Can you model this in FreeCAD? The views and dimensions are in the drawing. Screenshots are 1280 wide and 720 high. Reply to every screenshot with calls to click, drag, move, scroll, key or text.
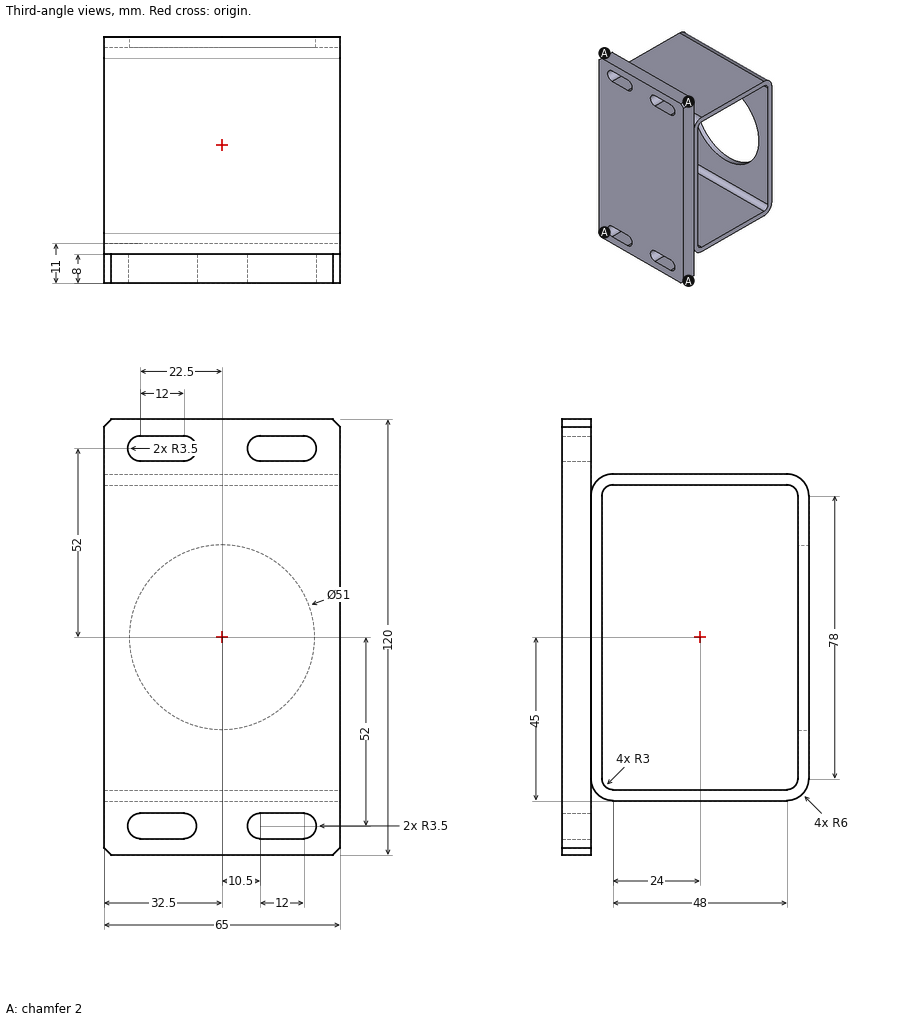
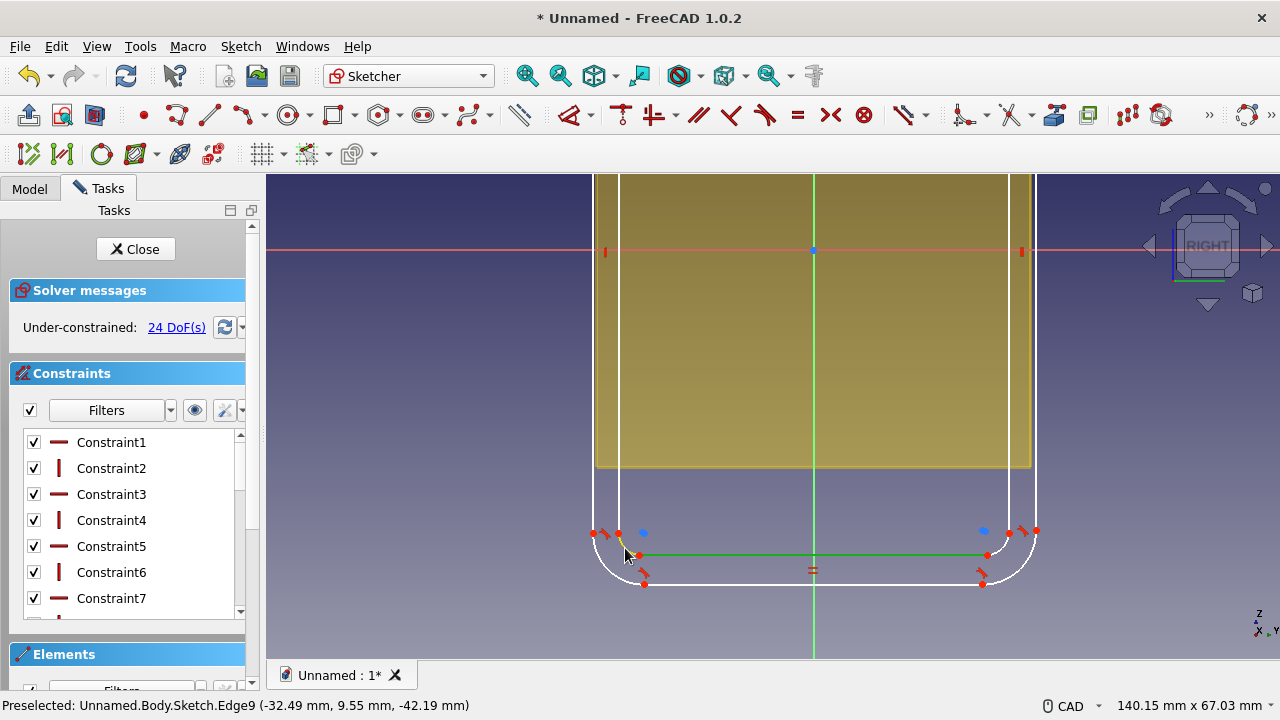
click(625, 548)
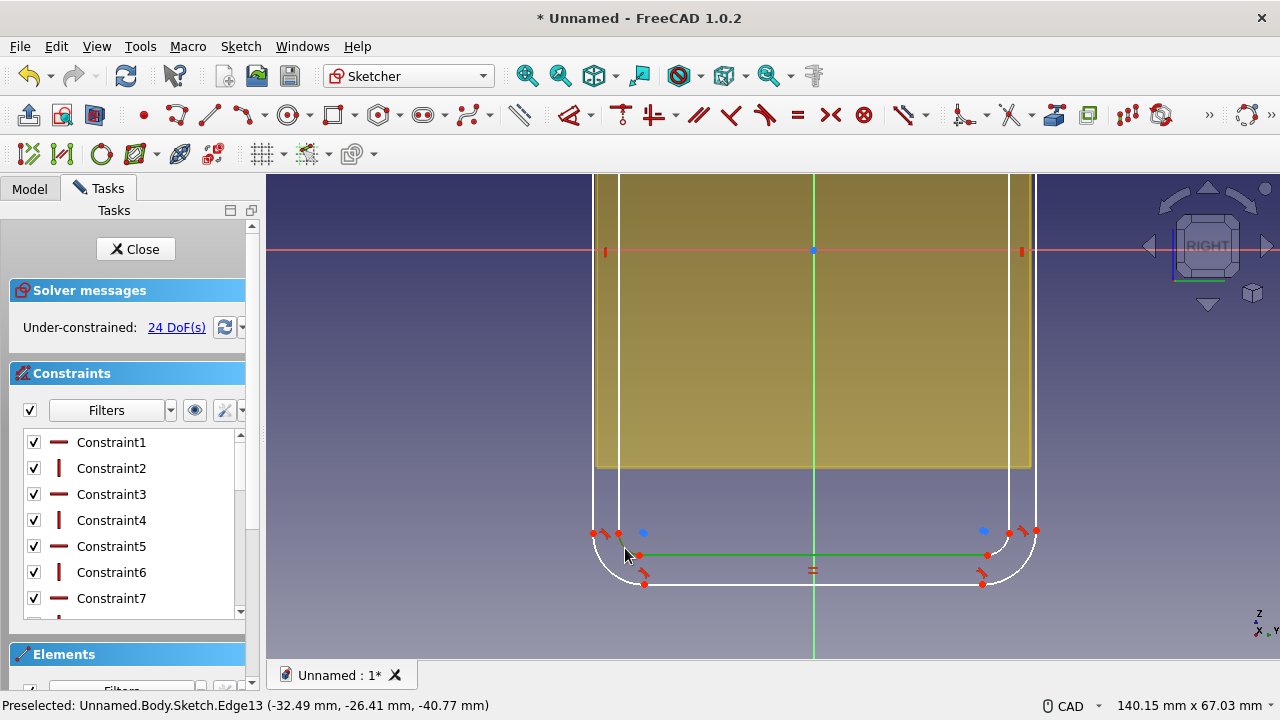
click(765, 116)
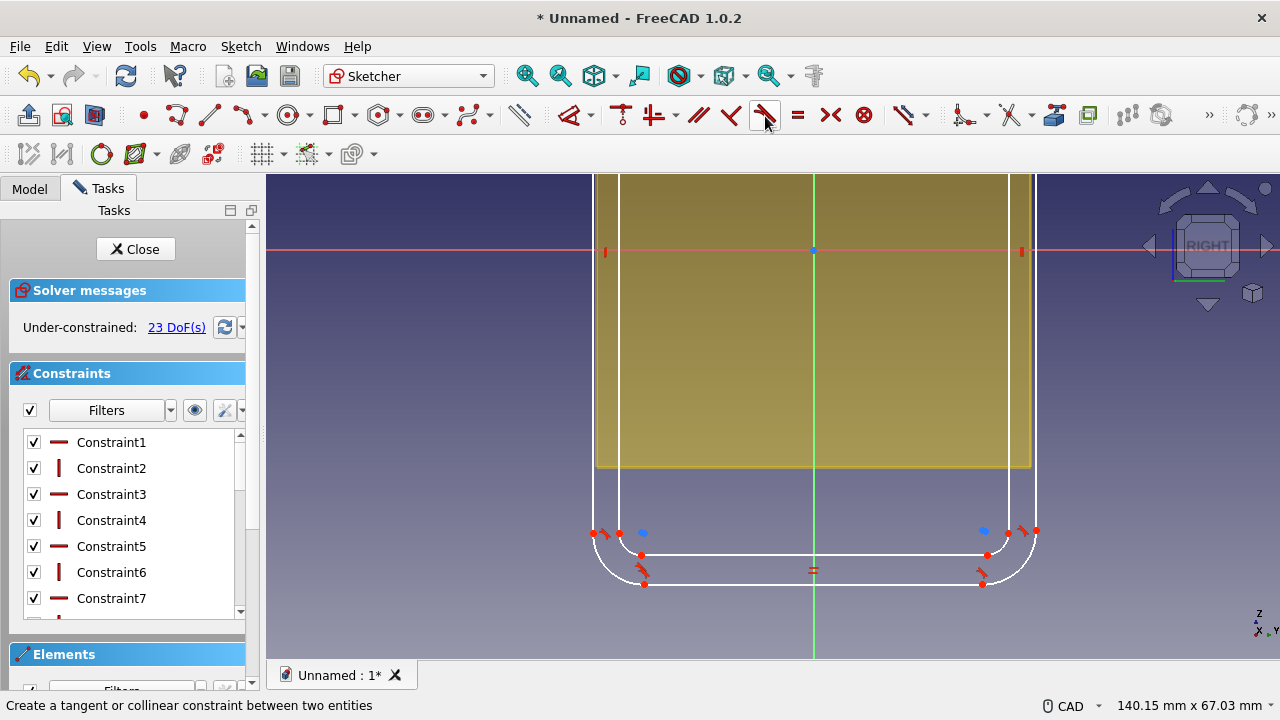
click(884, 555)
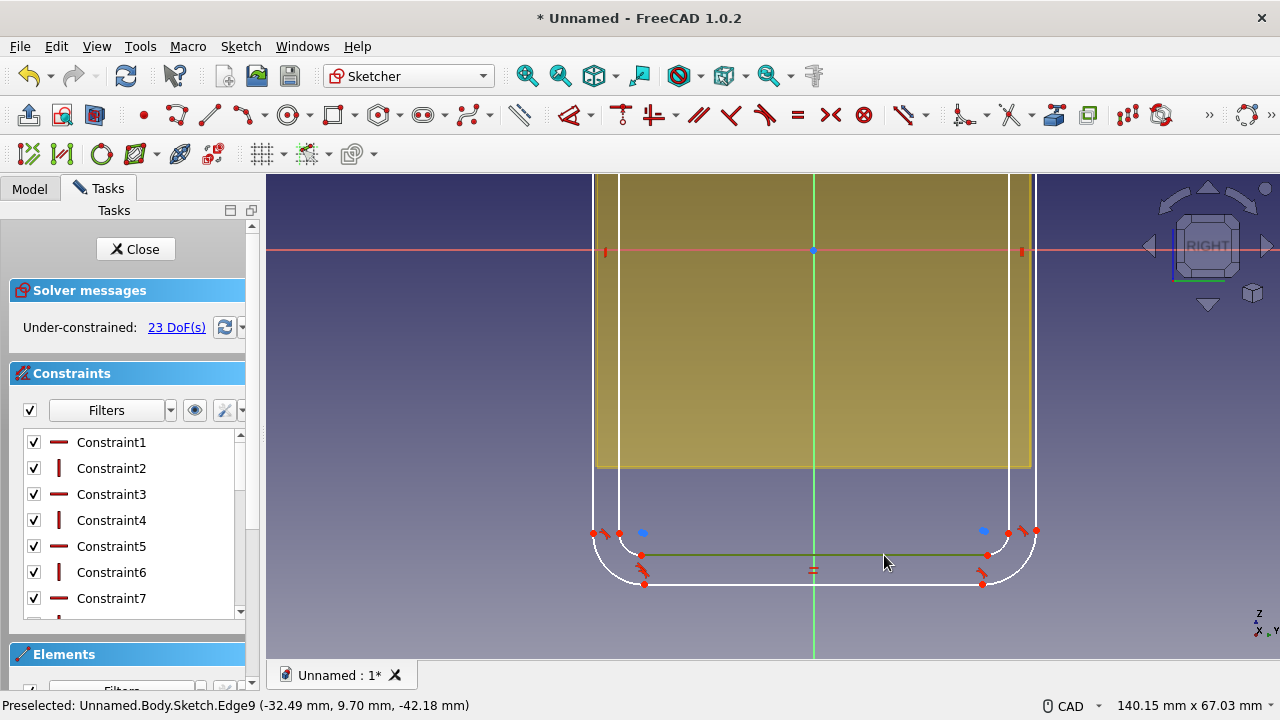
scroll(997, 552, up, 2)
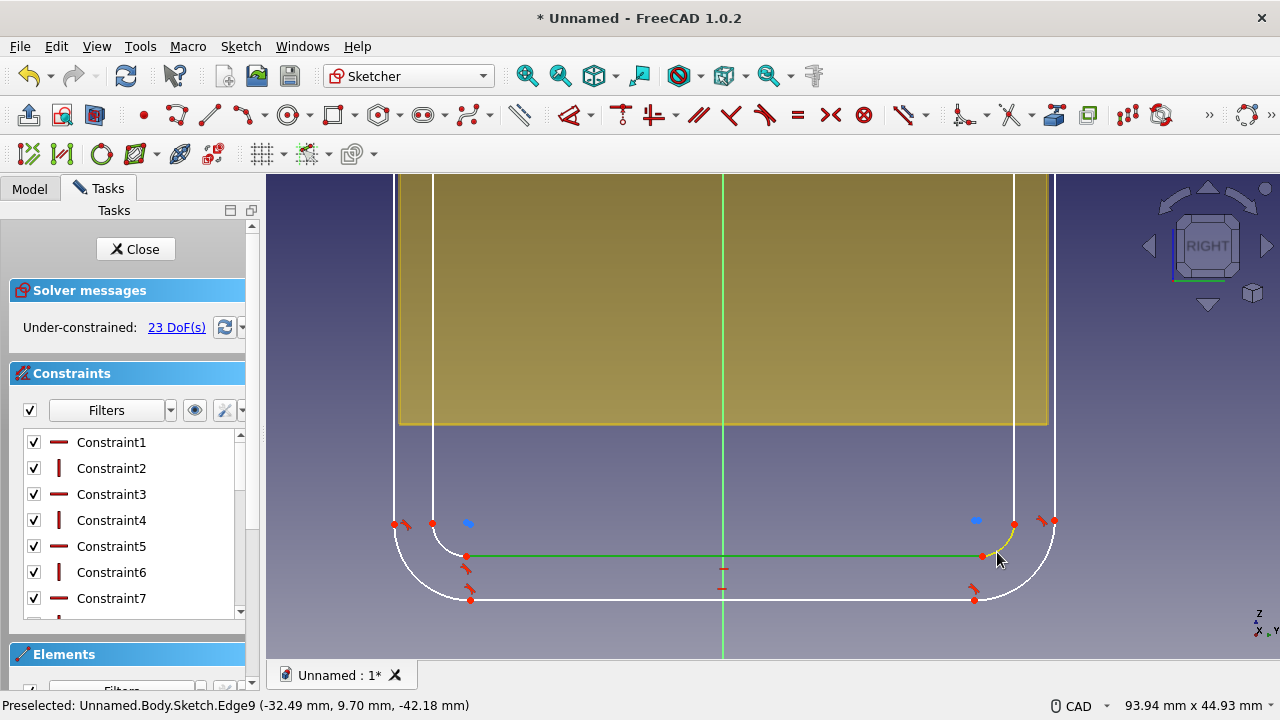
click(997, 552)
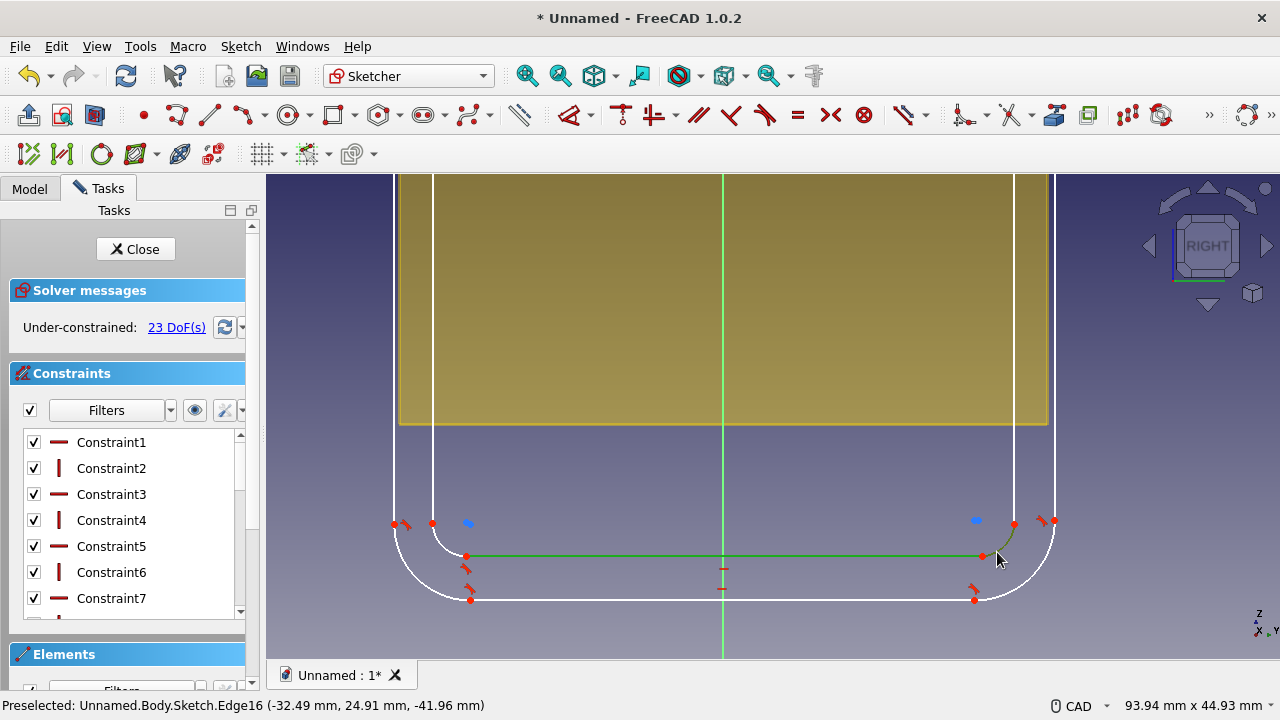
click(765, 116)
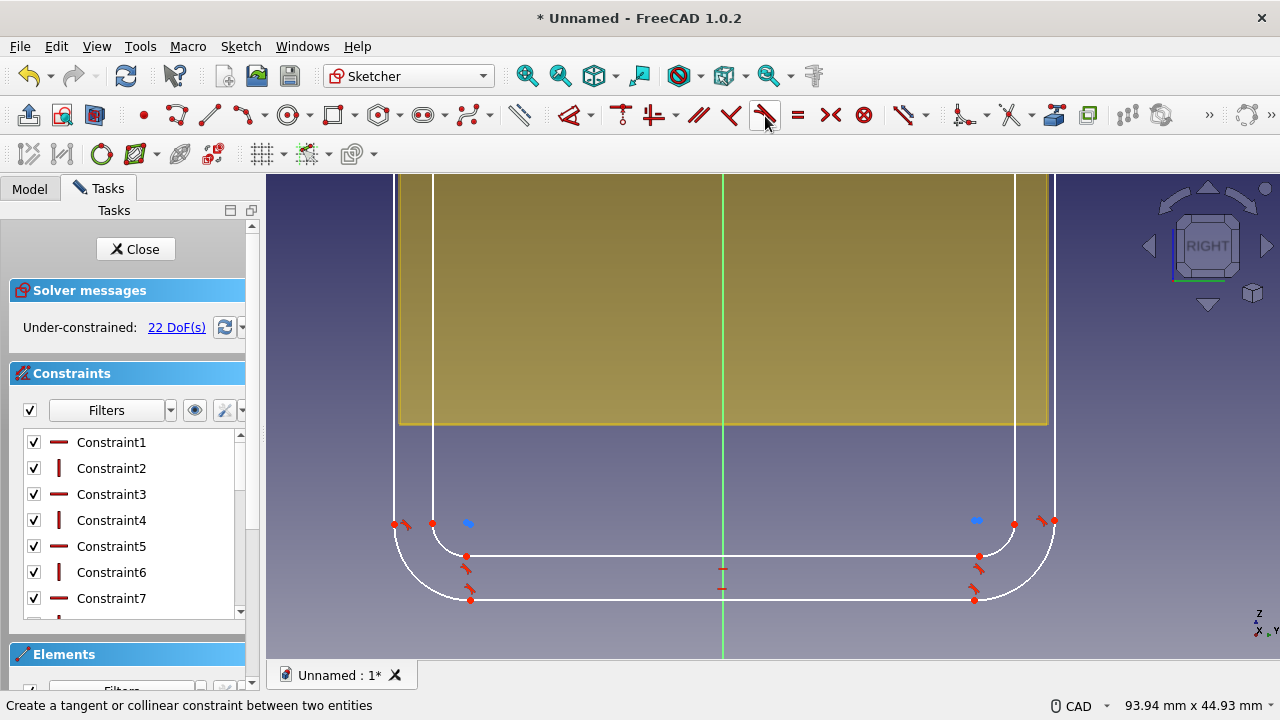
click(433, 271)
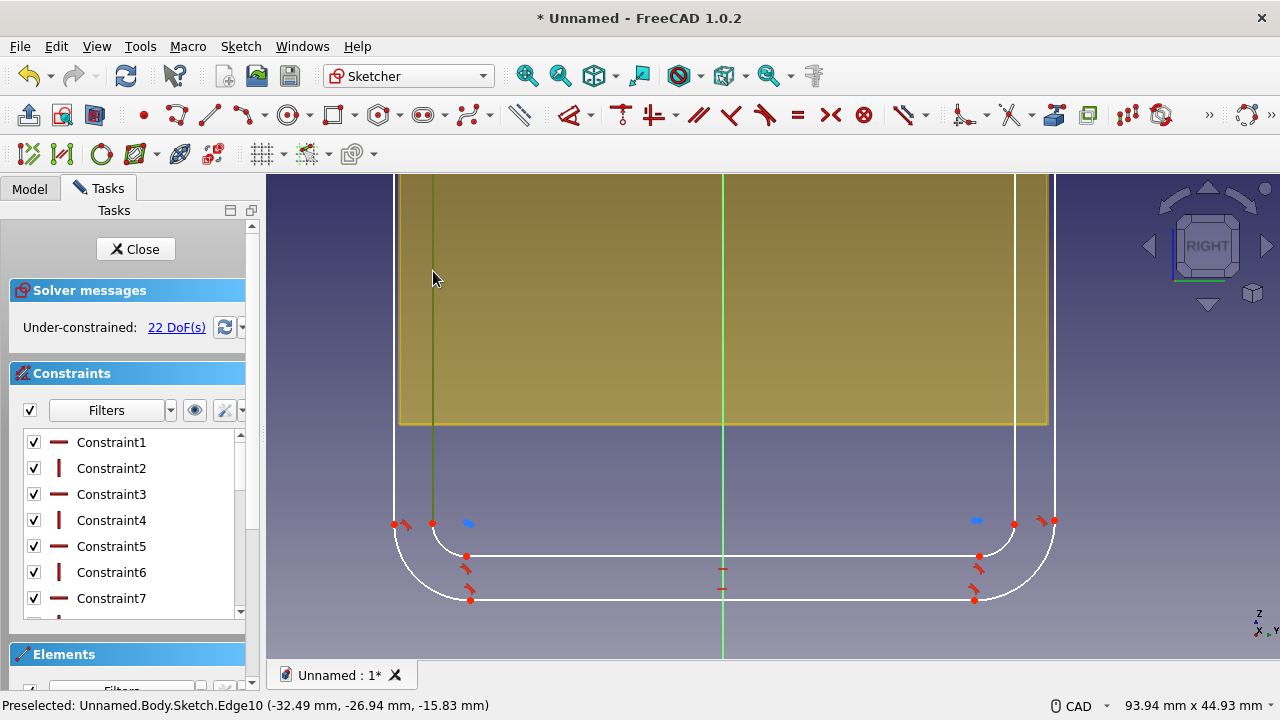
click(437, 539)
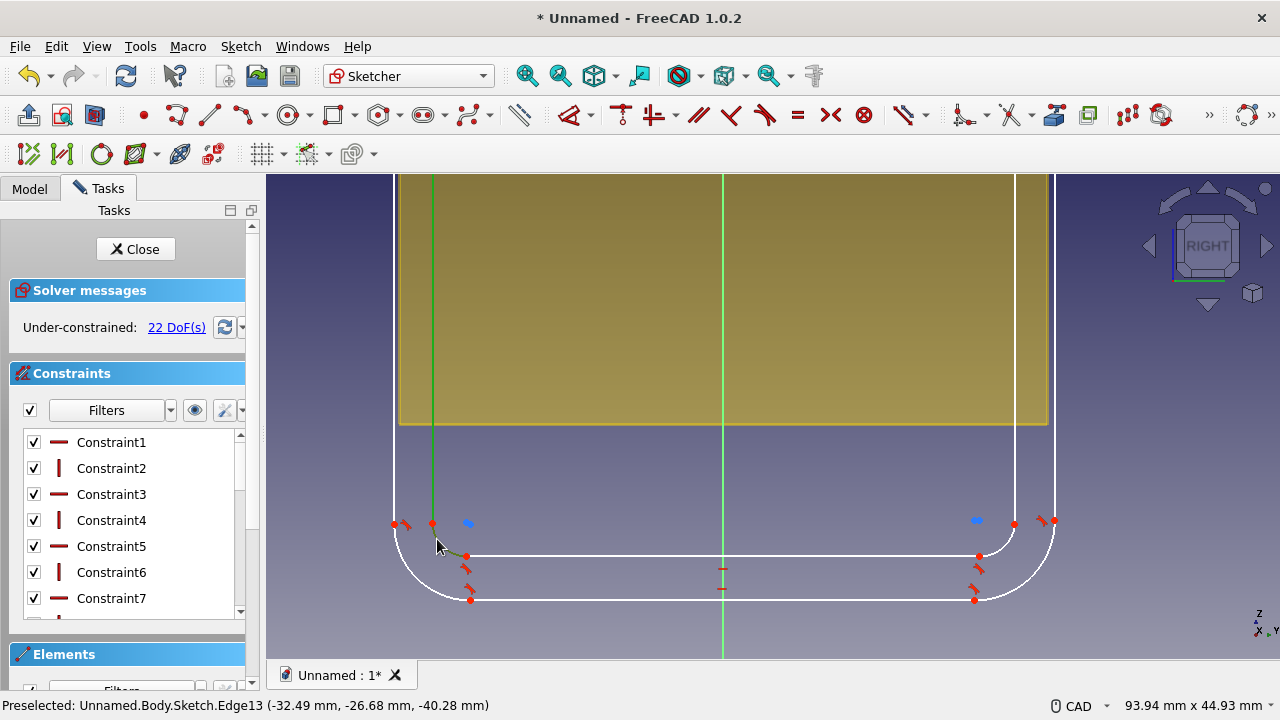
click(765, 116)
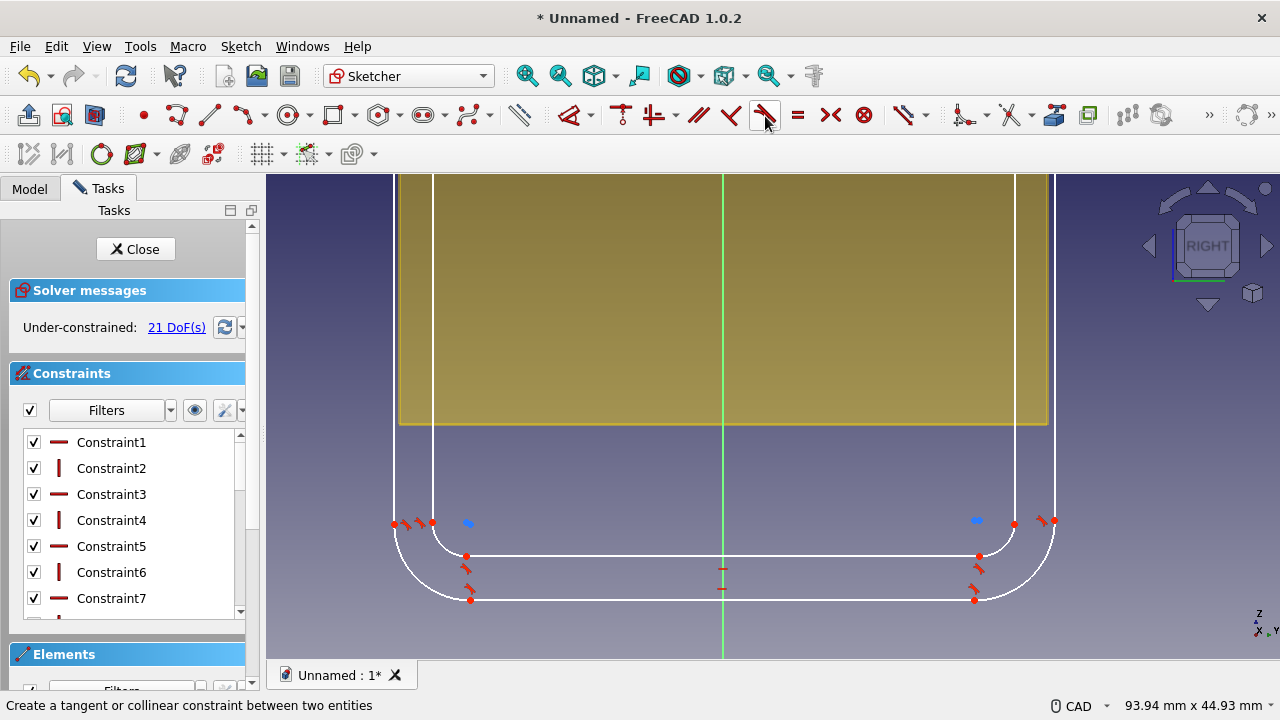
click(433, 270)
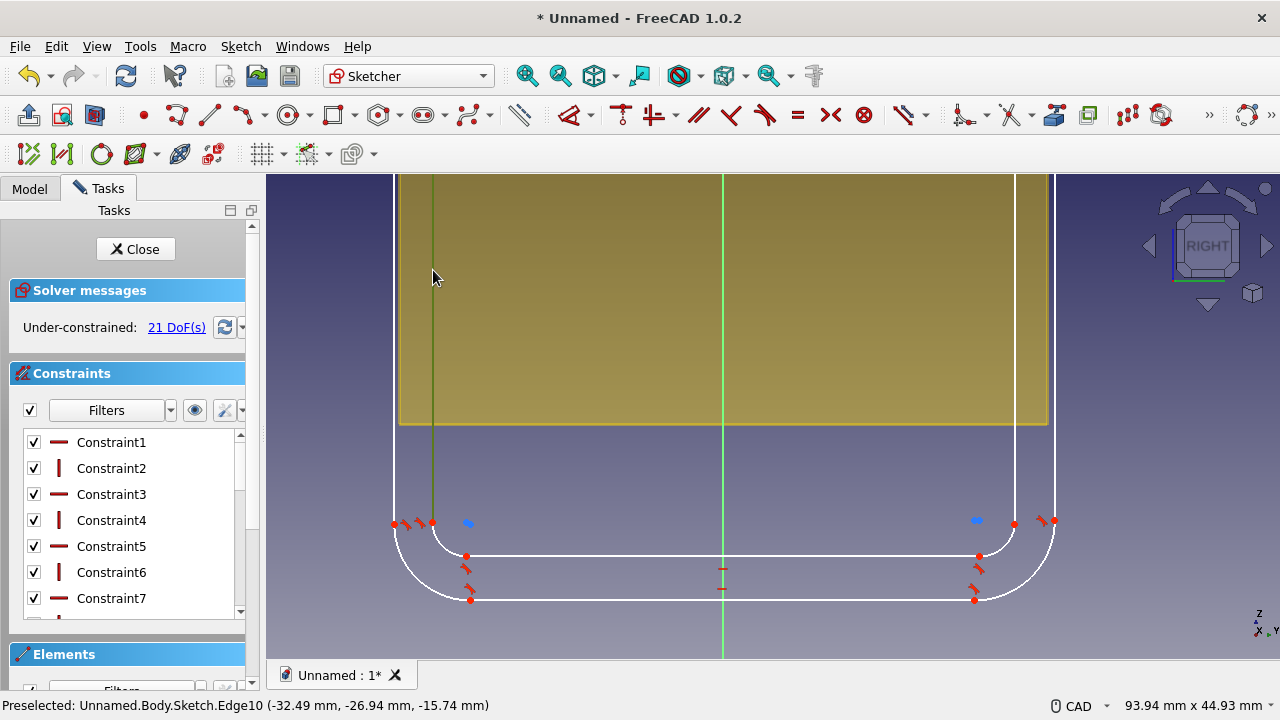
scroll(696, 552, down, 6)